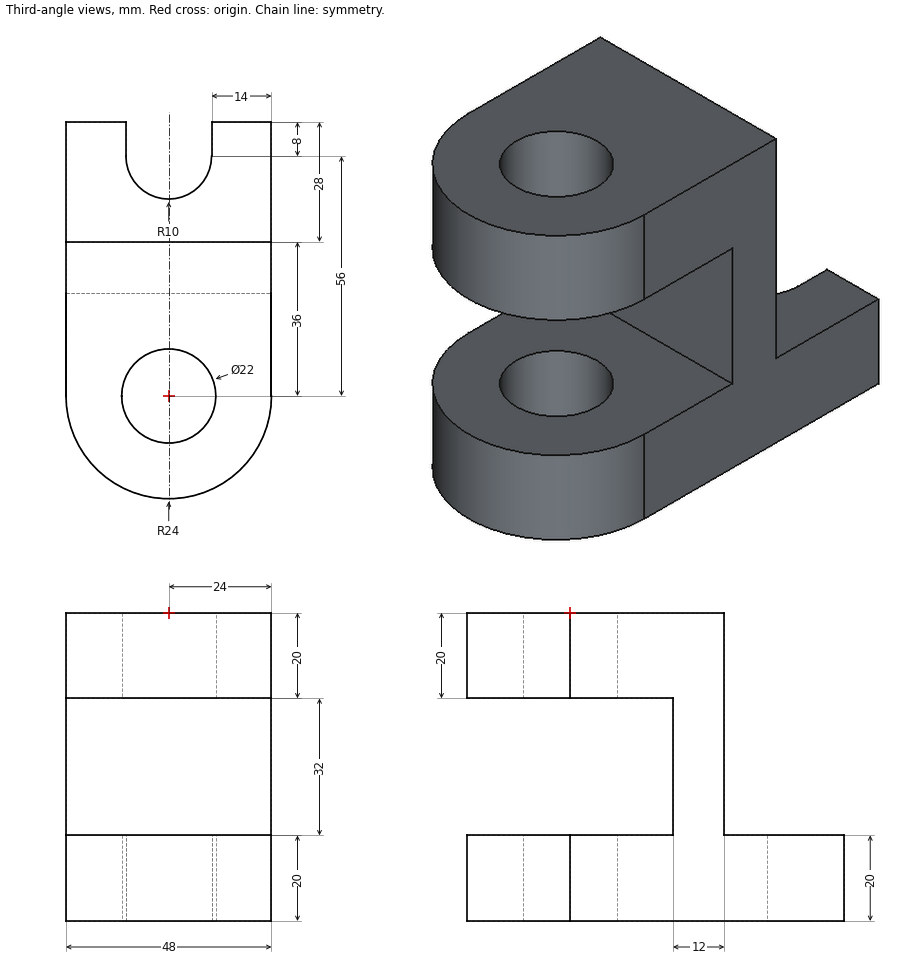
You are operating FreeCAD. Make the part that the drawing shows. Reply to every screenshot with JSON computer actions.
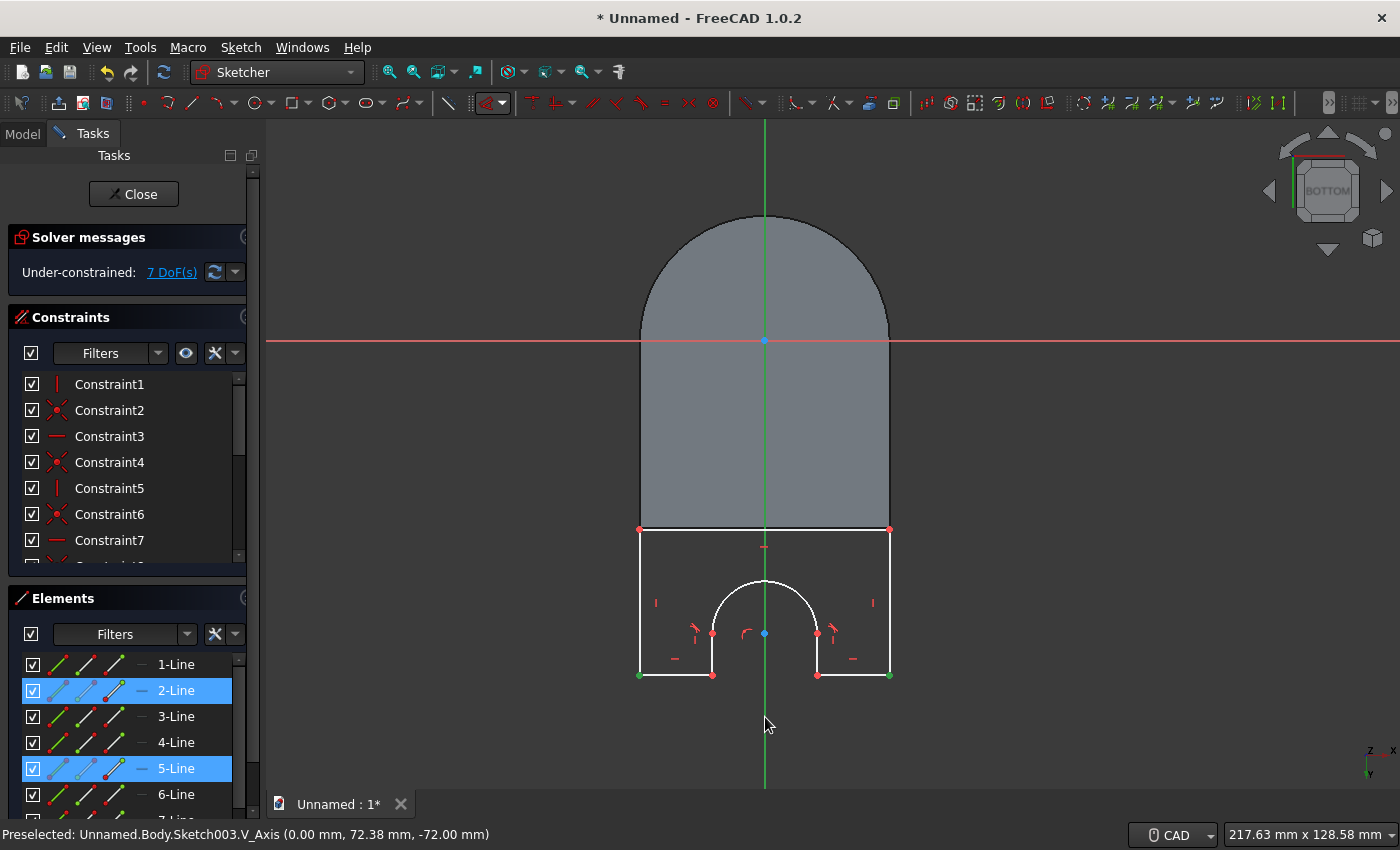
{"action": "left_click", "coordinate": [690, 104]}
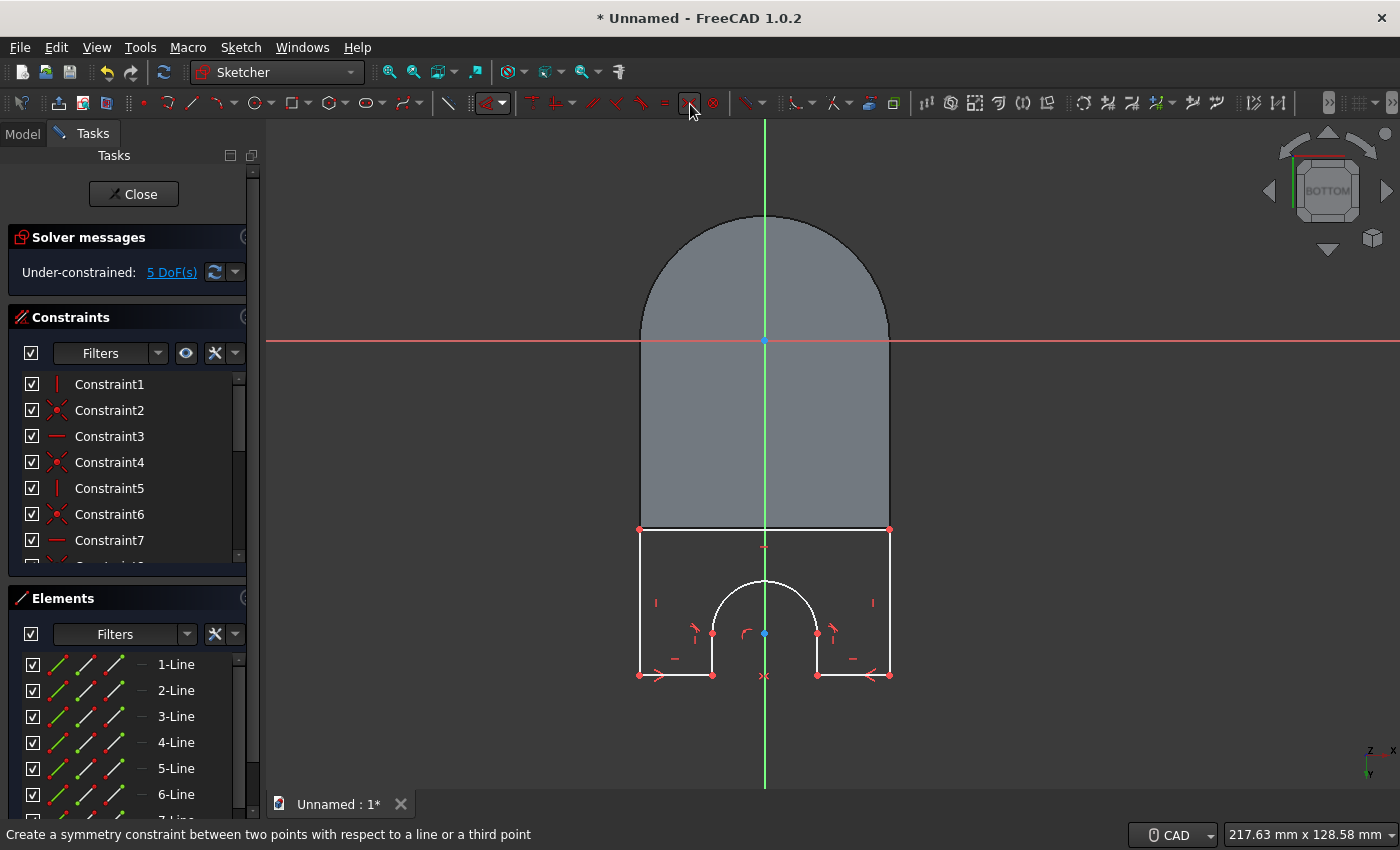
{"action": "left_click", "coordinate": [795, 591]}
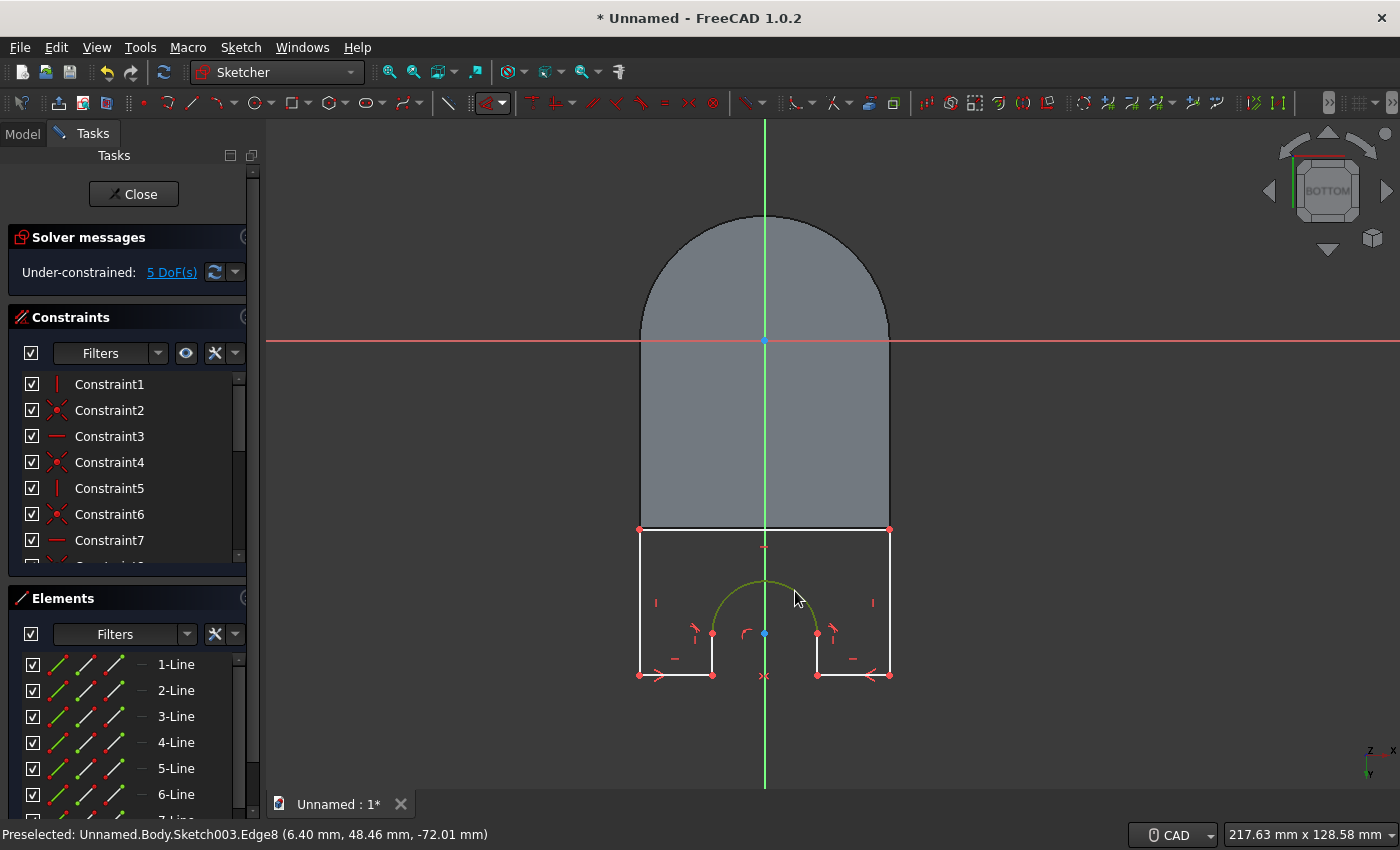
{"action": "left_click", "coordinate": [504, 104]}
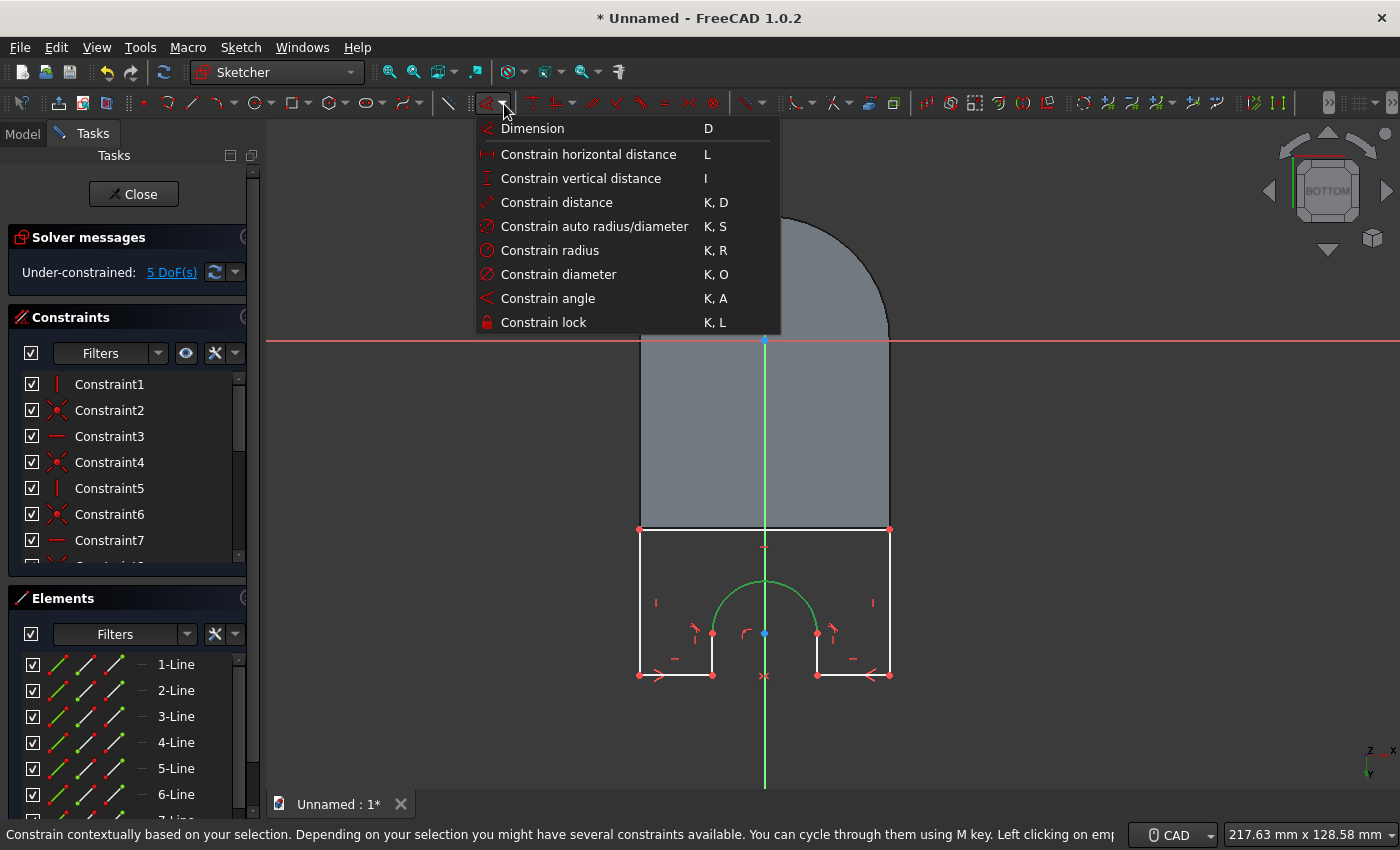
{"action": "left_click", "coordinate": [628, 250]}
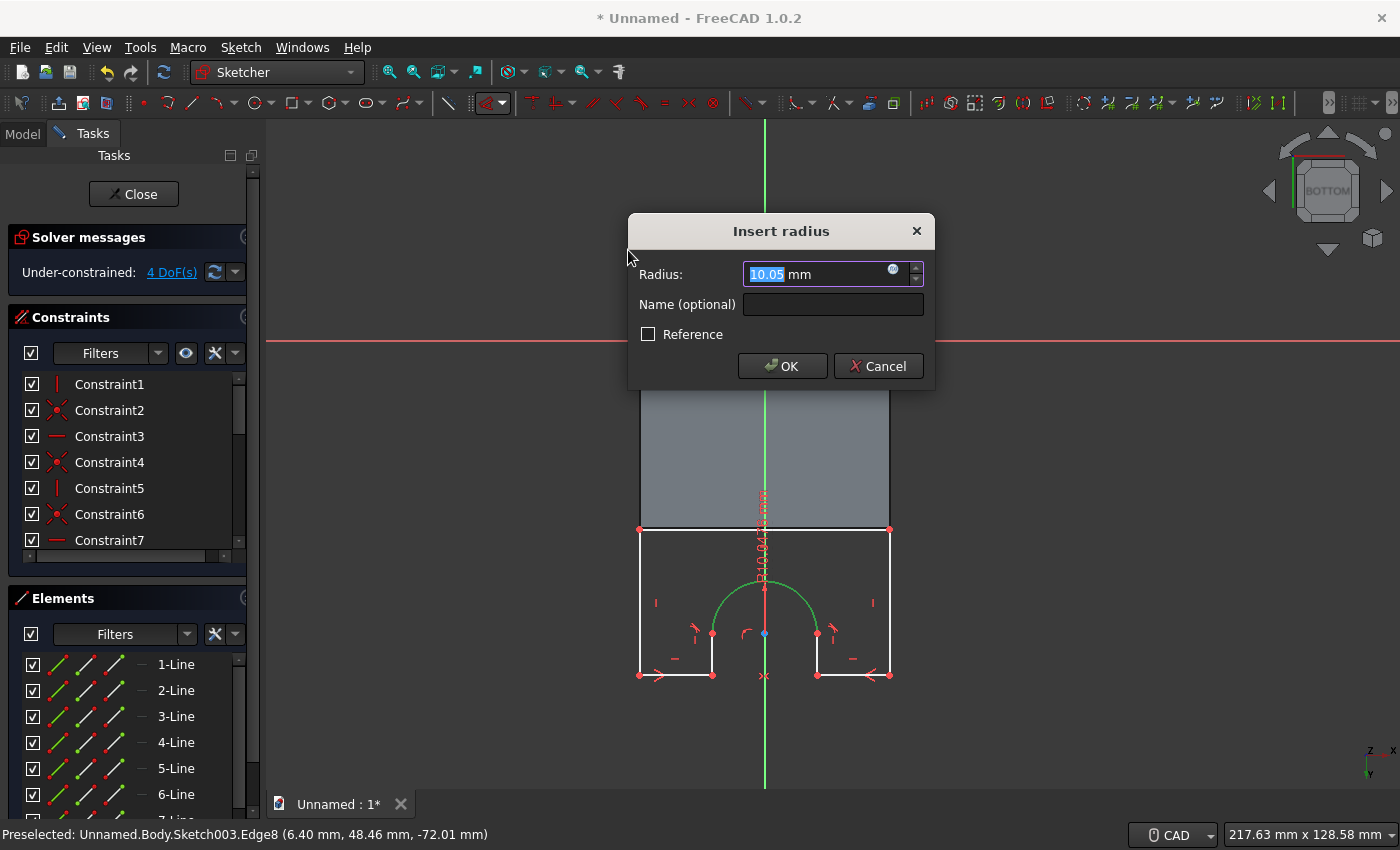
{"action": "type", "text": "10"}
{"action": "key", "text": "Return"}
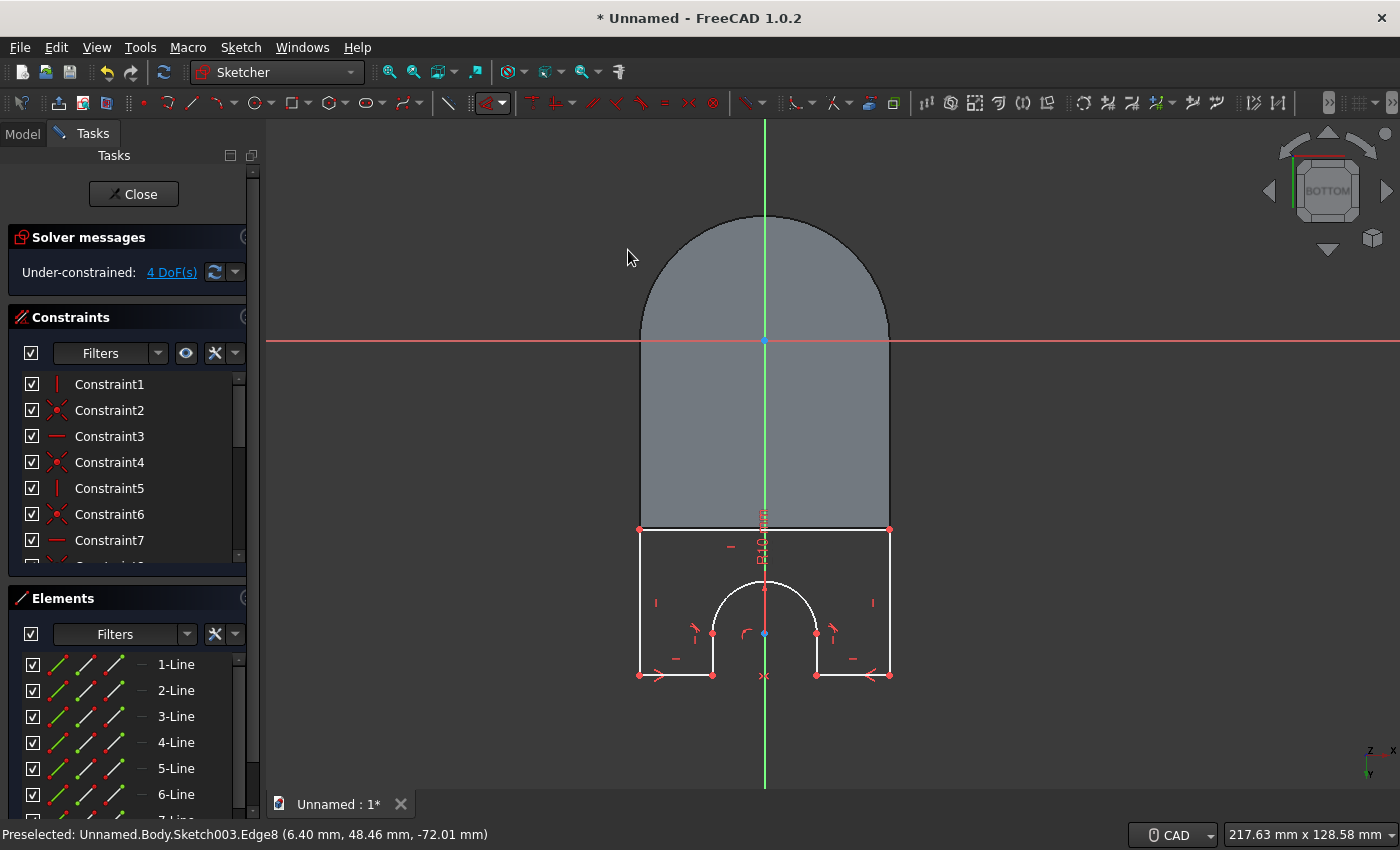
{"action": "left_click", "coordinate": [817, 646]}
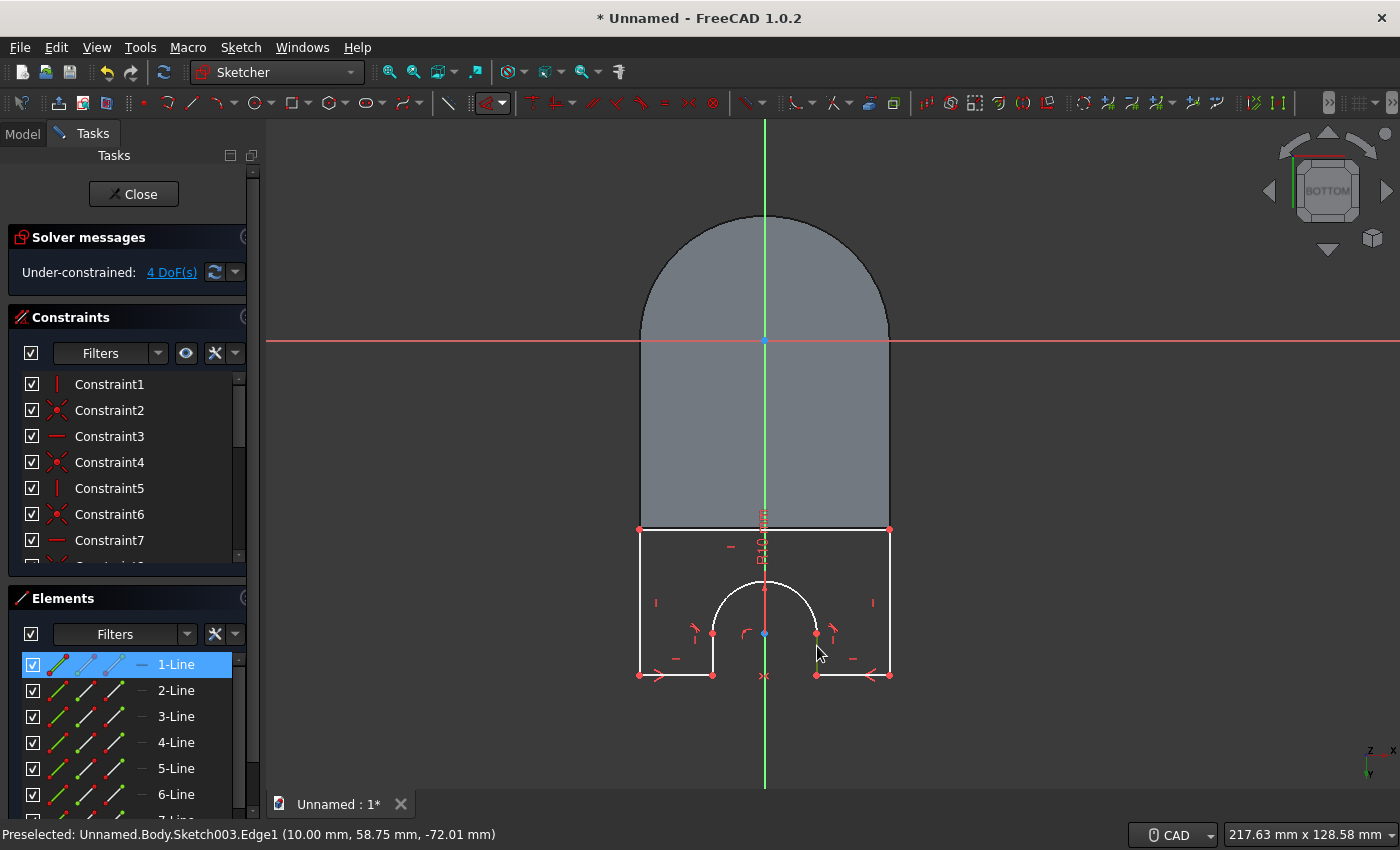
{"action": "left_click", "coordinate": [504, 104]}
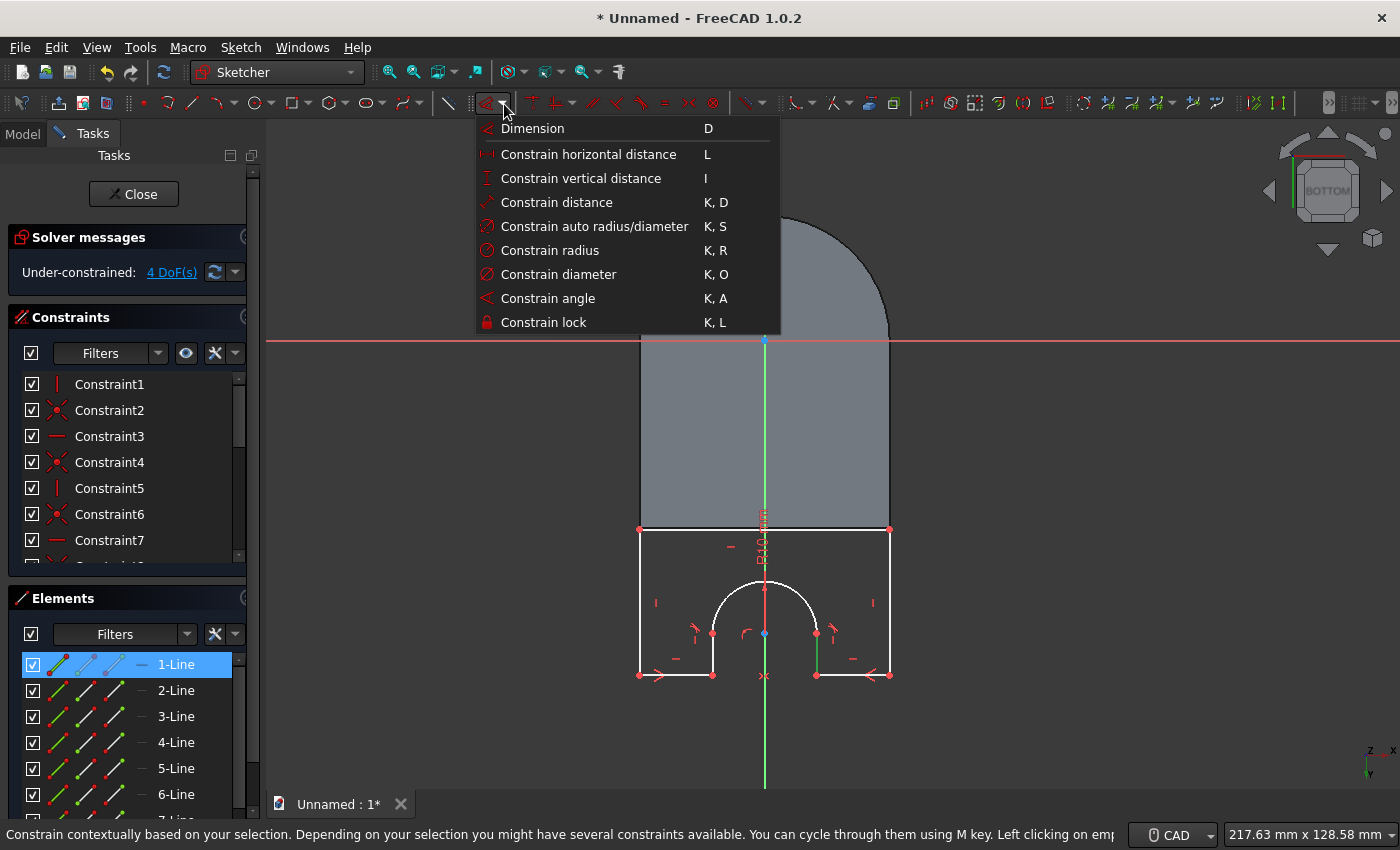
{"action": "left_click", "coordinate": [628, 178]}